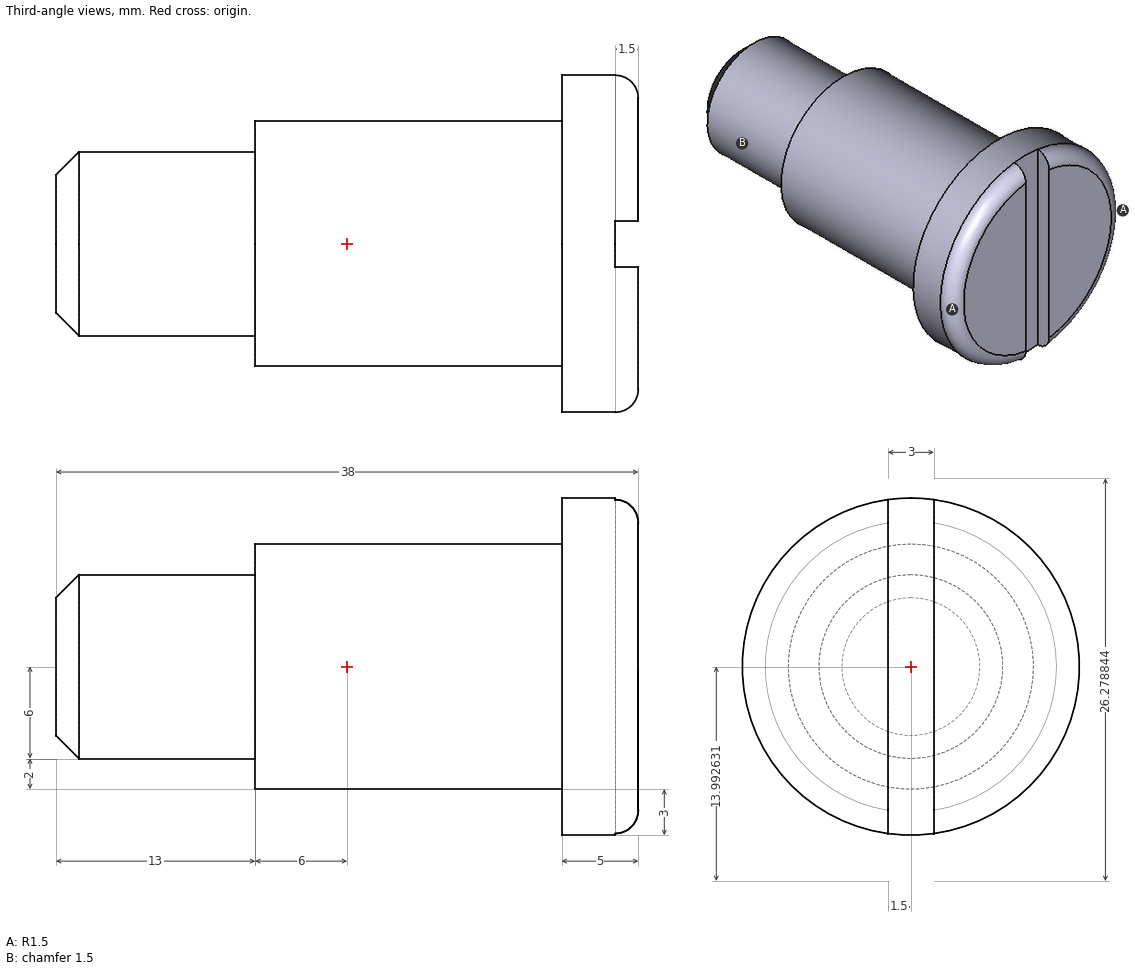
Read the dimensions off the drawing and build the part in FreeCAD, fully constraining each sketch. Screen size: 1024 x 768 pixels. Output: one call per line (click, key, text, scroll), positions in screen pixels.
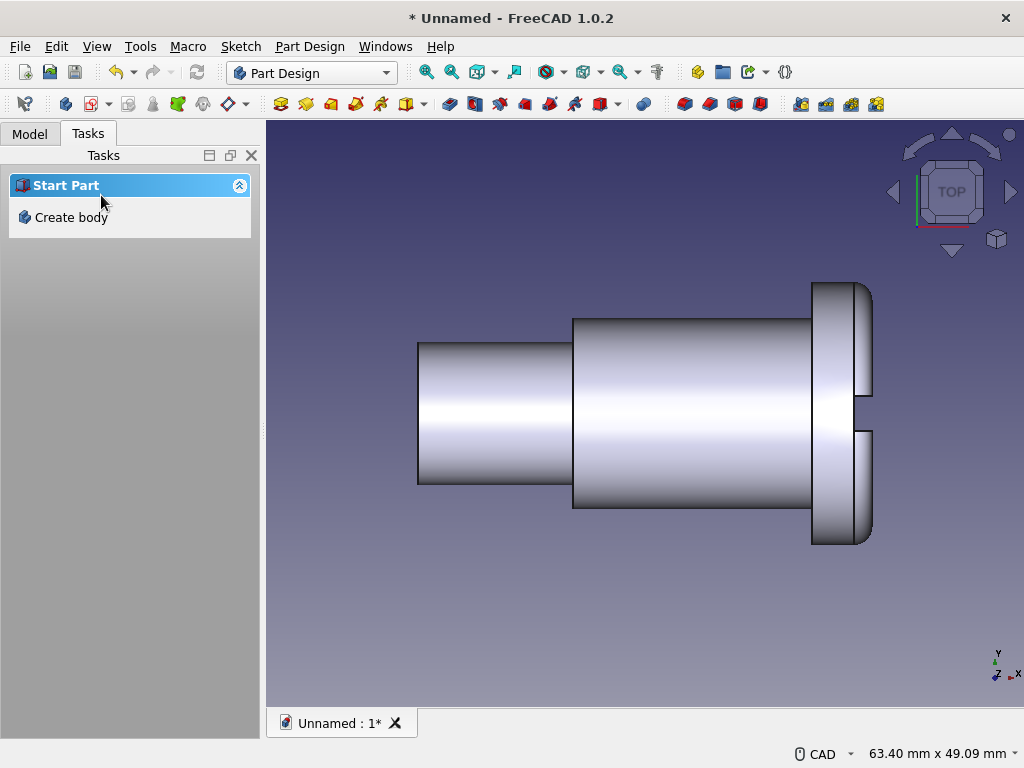
click(418, 412)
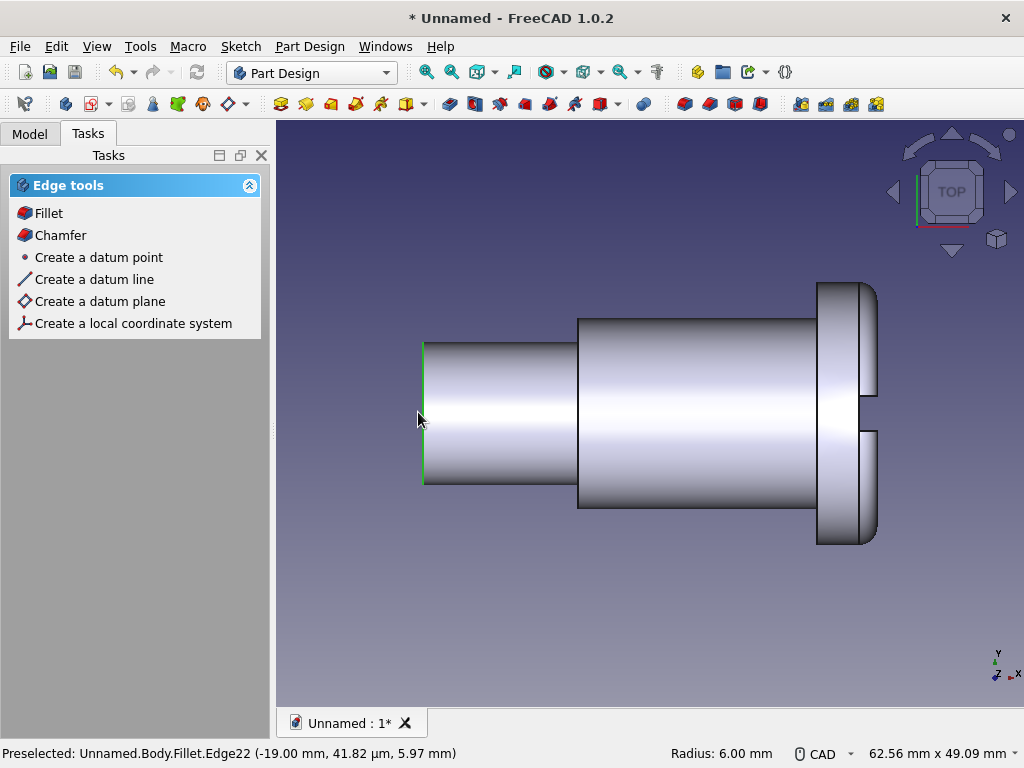
click(710, 104)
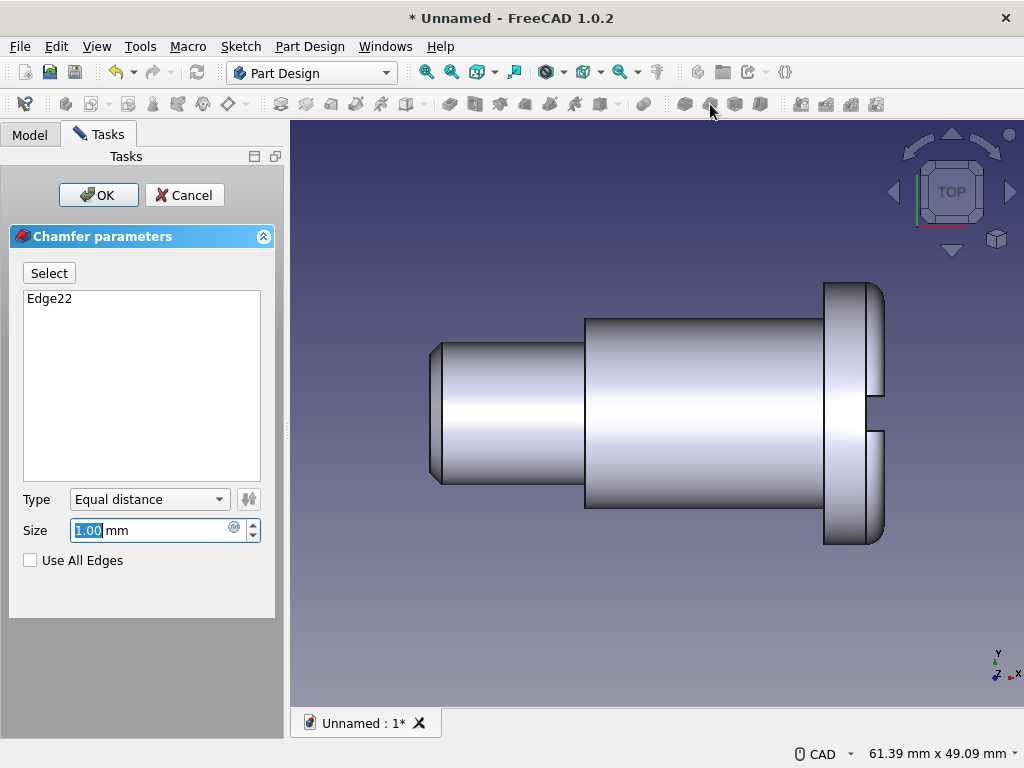
text(1.5)
key(Tab)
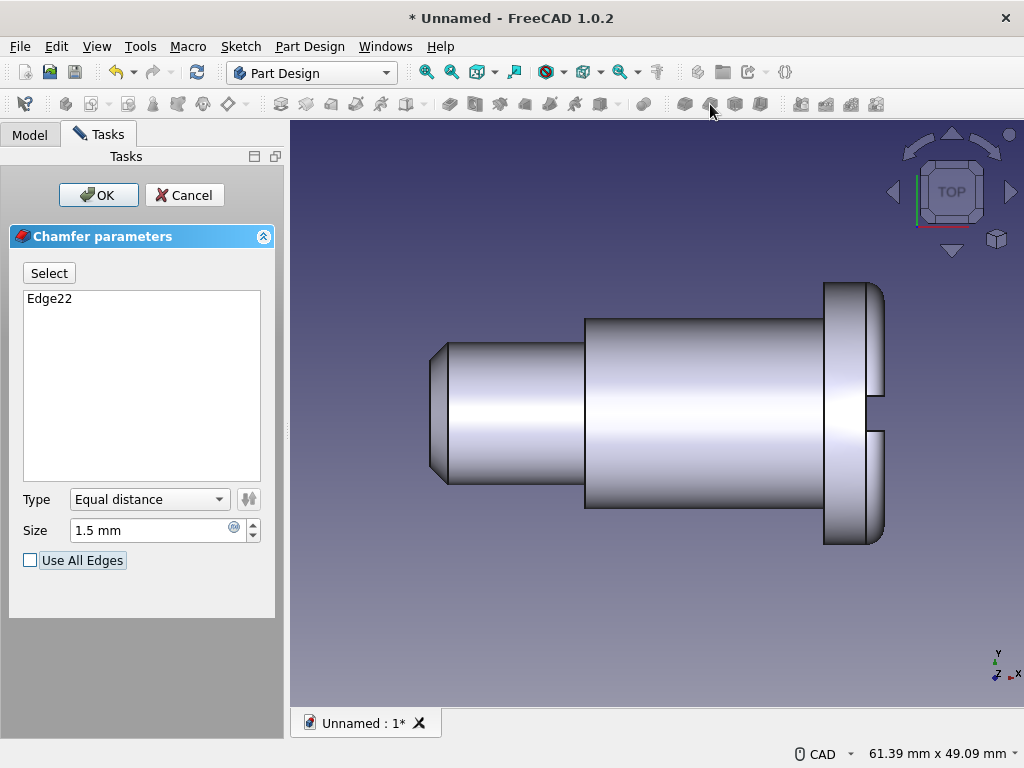
click(99, 195)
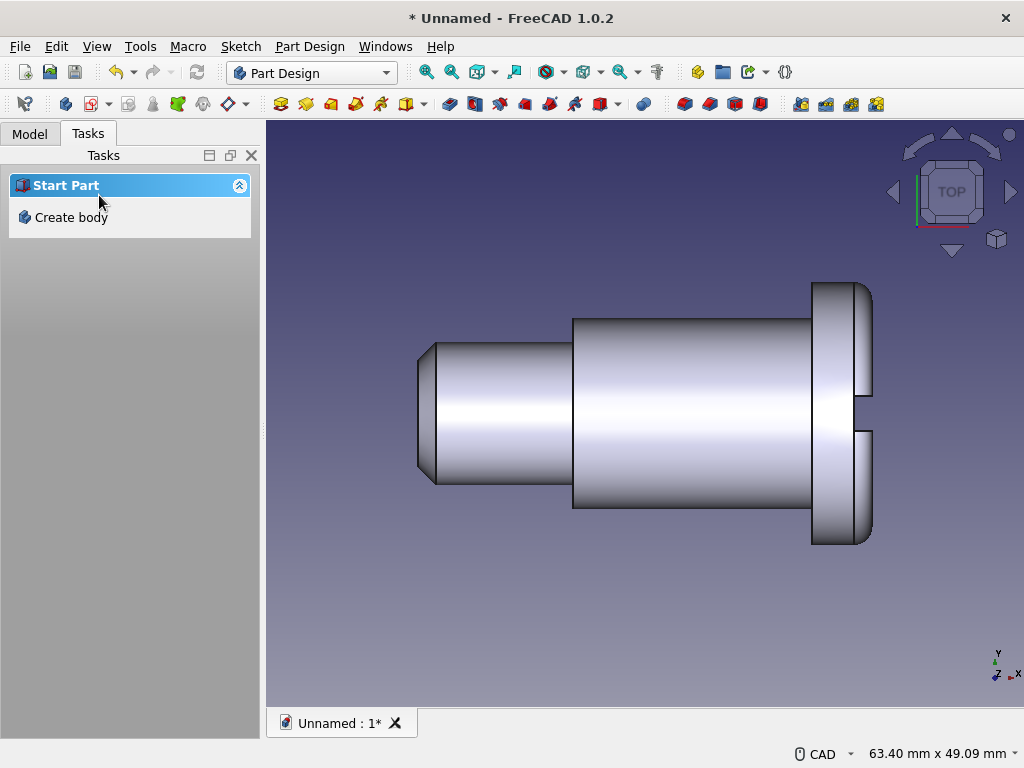
key(0)